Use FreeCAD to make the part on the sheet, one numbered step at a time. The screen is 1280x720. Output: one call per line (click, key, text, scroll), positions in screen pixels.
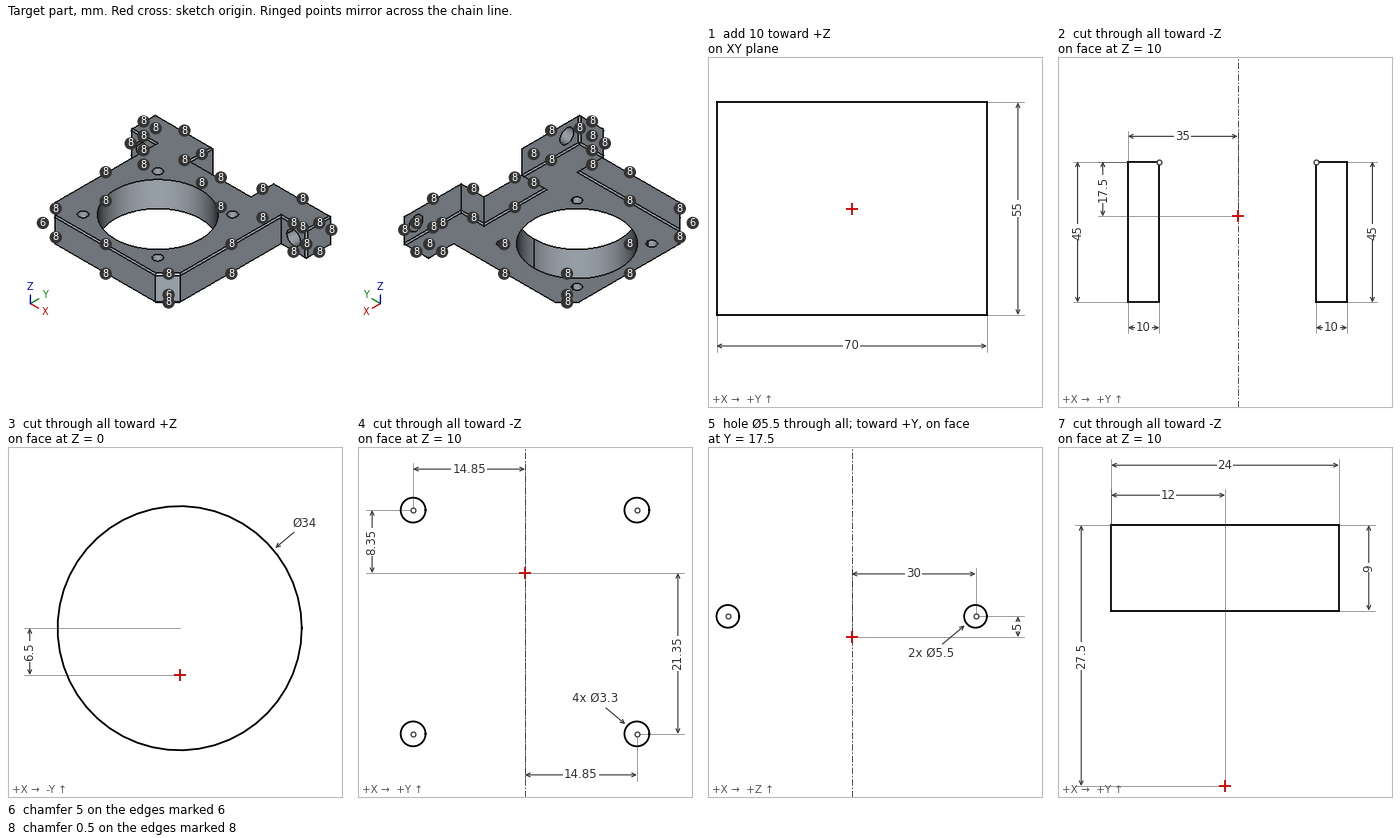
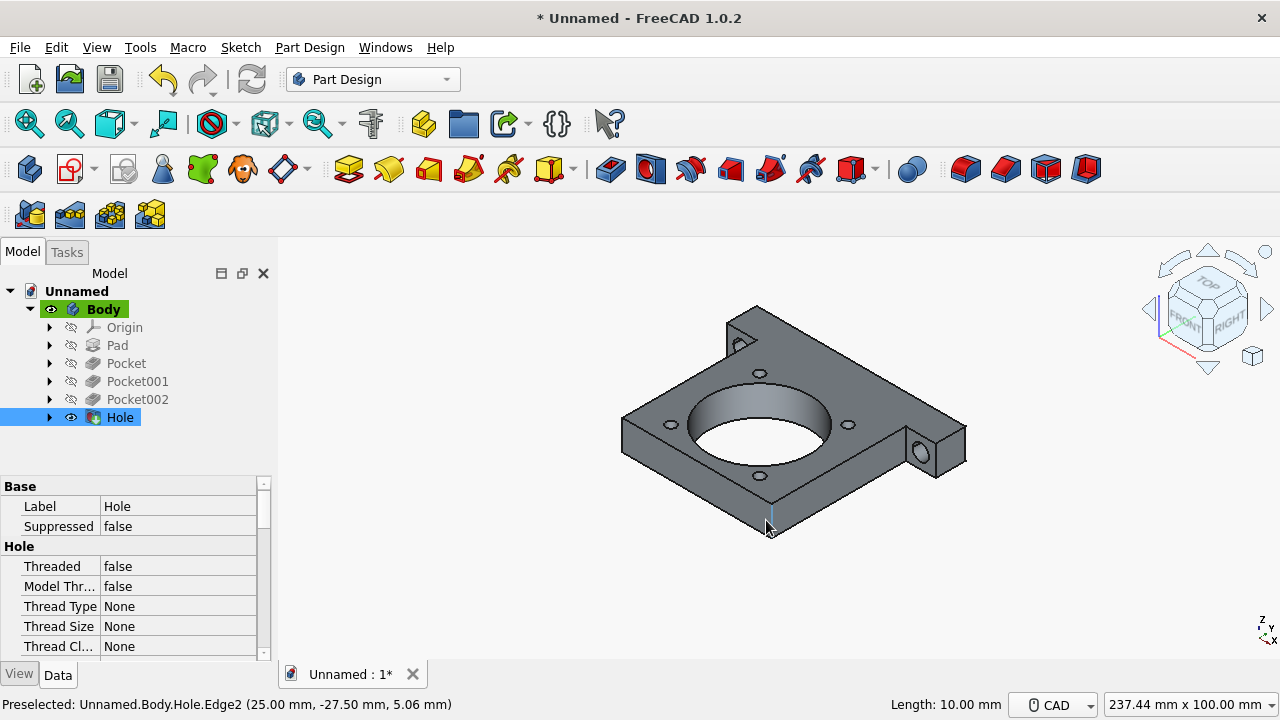
key(v)
key(f)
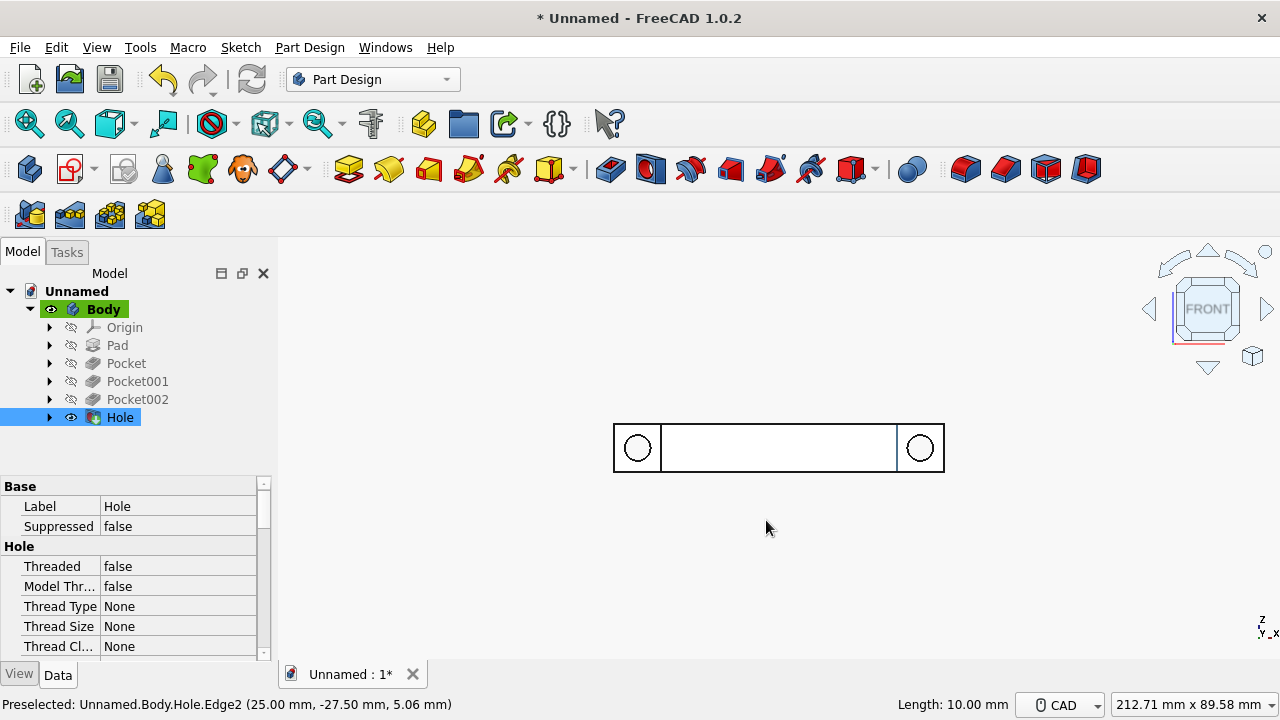
click(661, 447, ctrl)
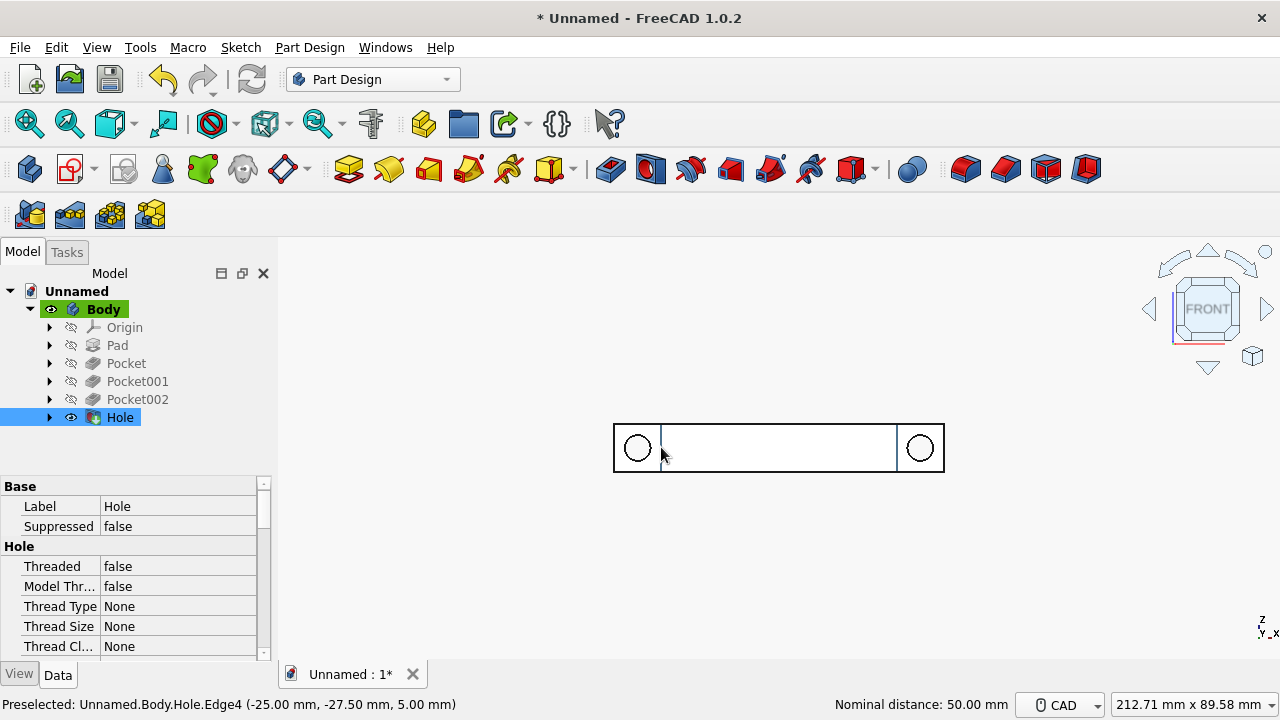
click(1006, 170)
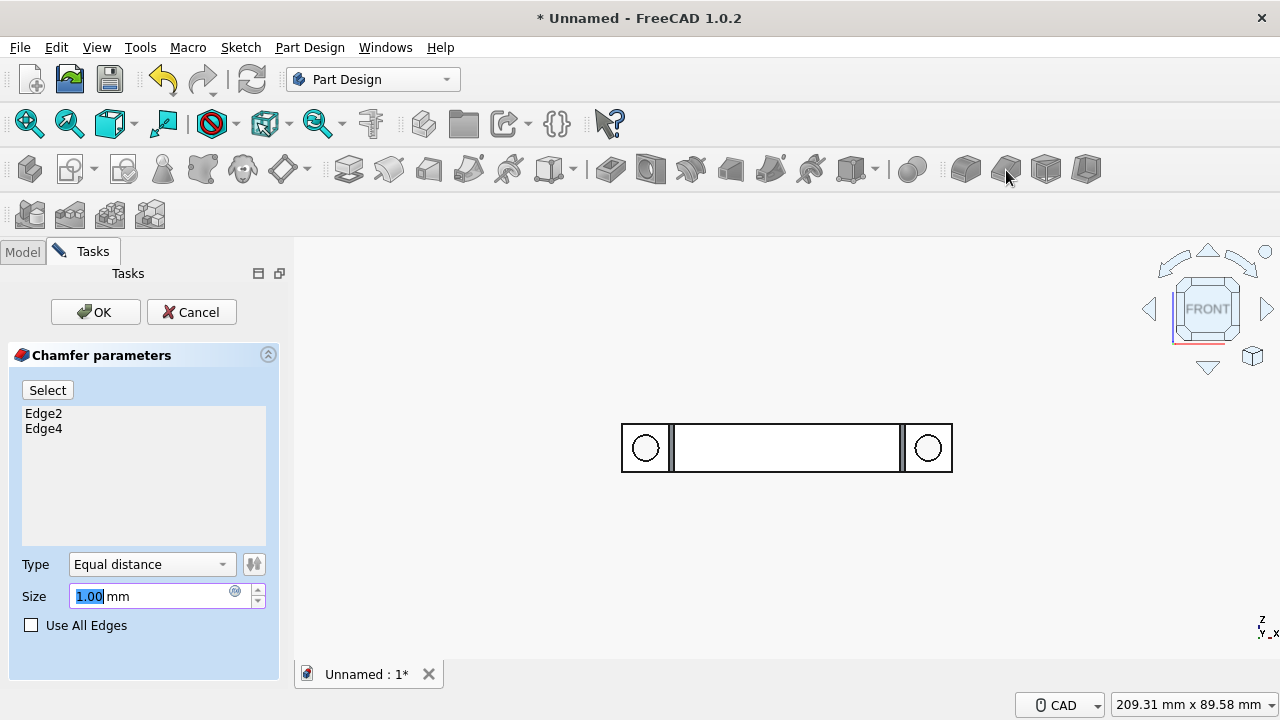
text(5)
key(Tab)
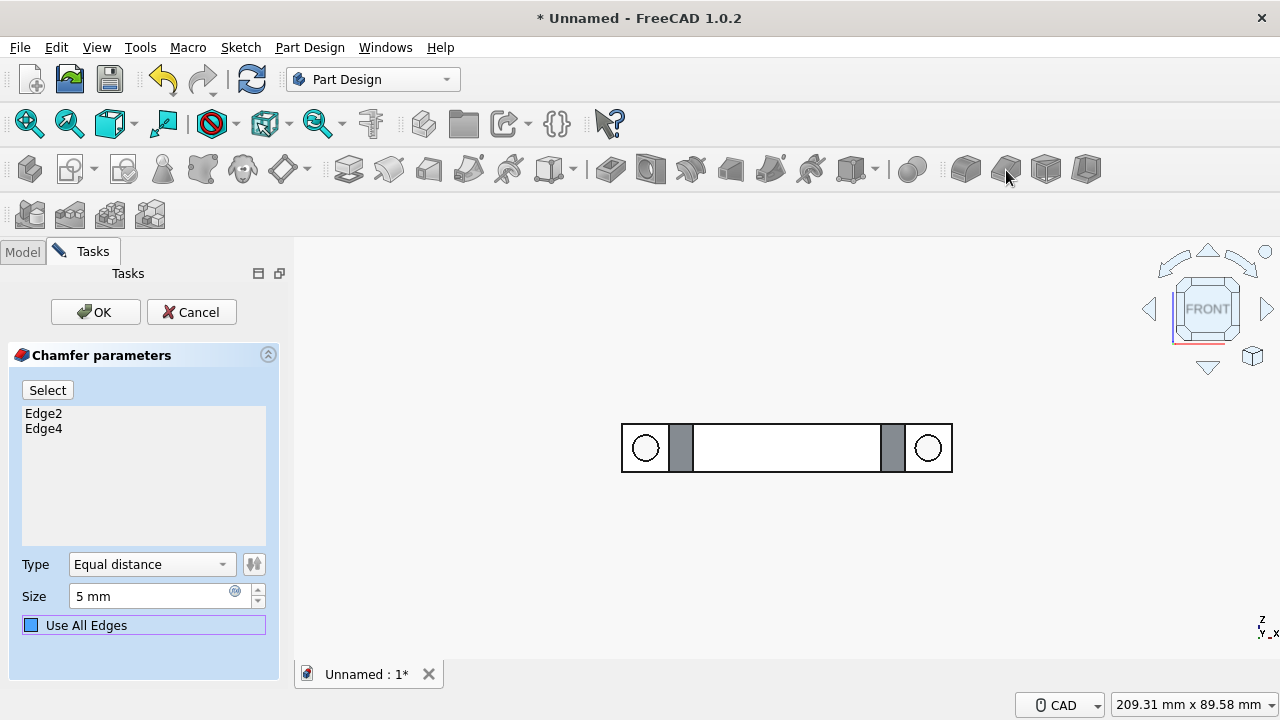
click(96, 312)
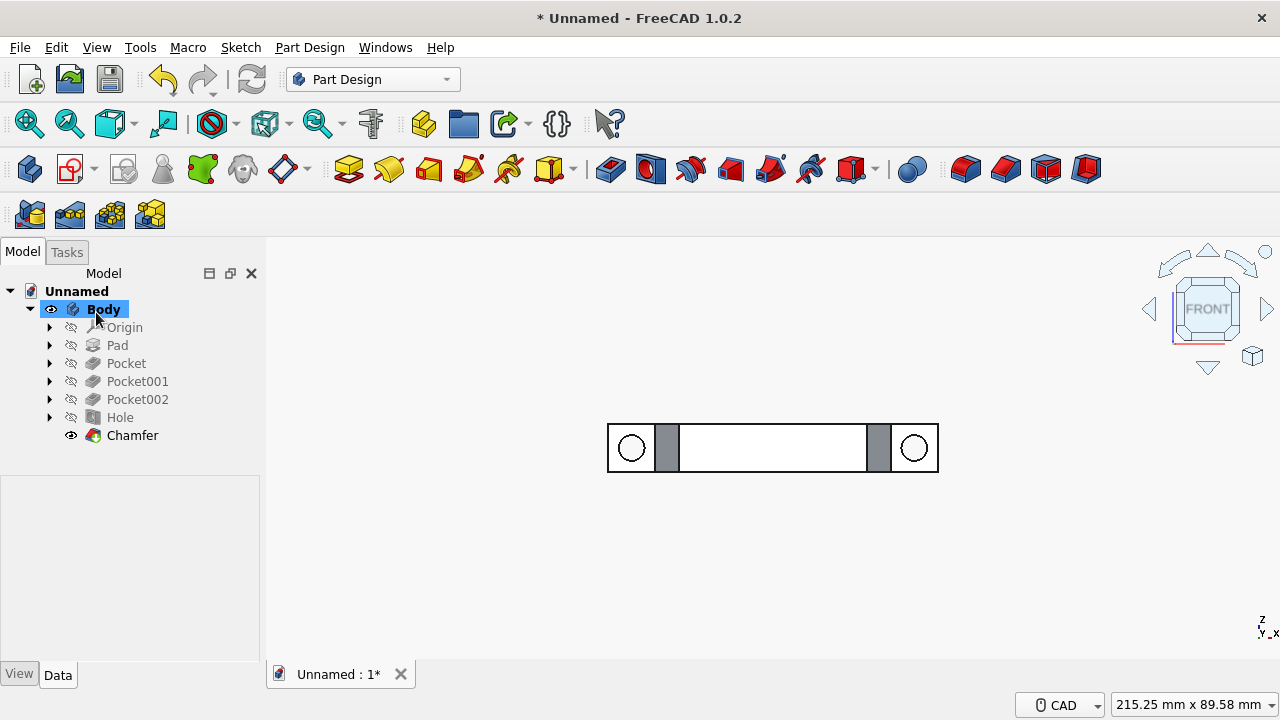
key(v)
key(f)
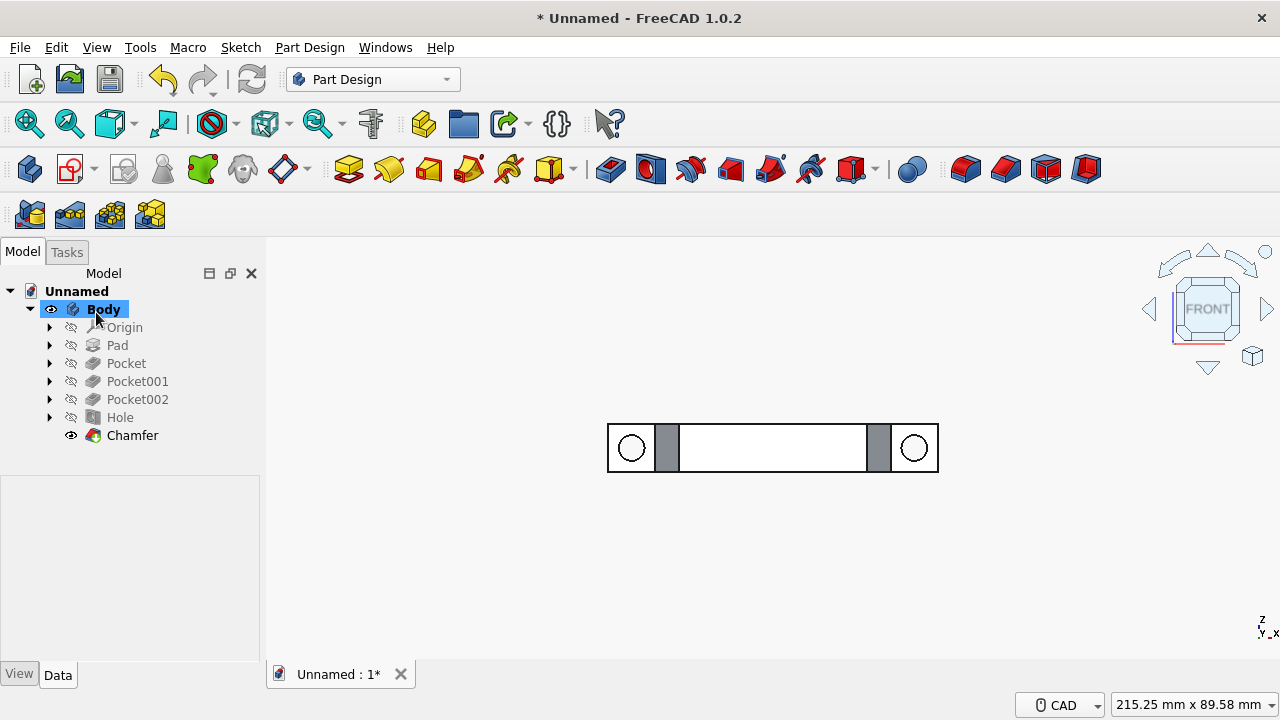
key(0)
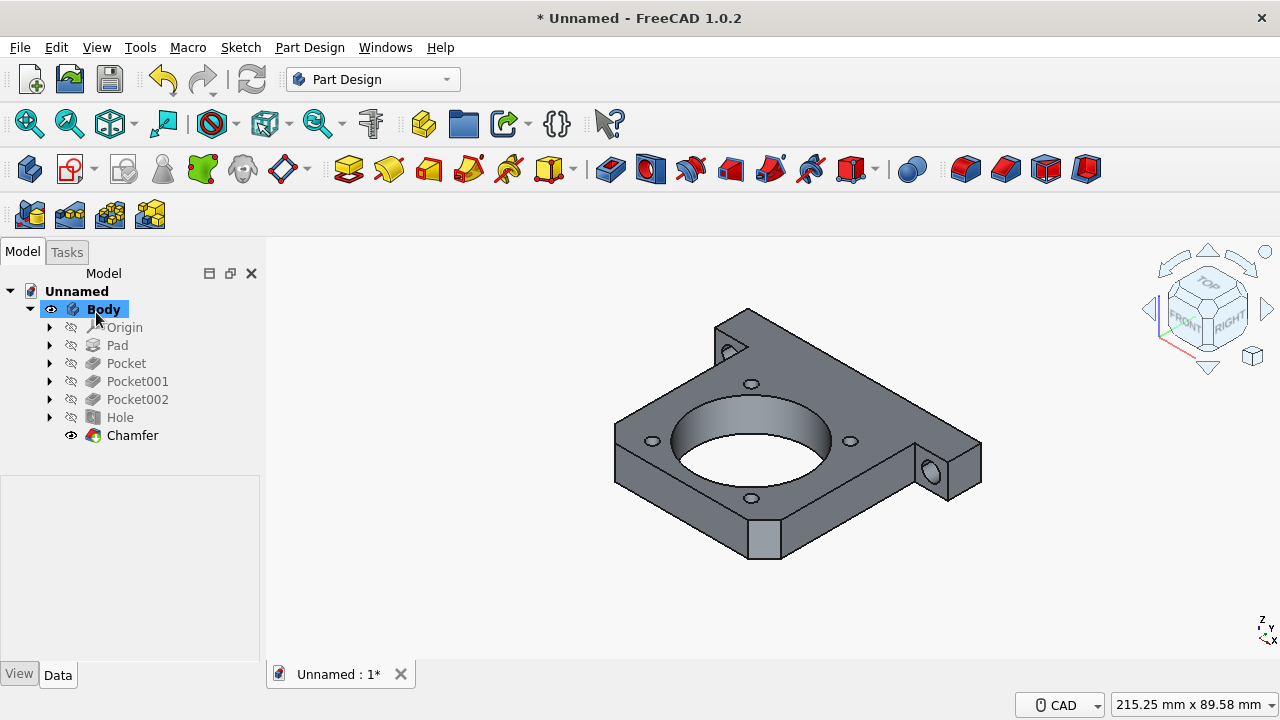
click(859, 417)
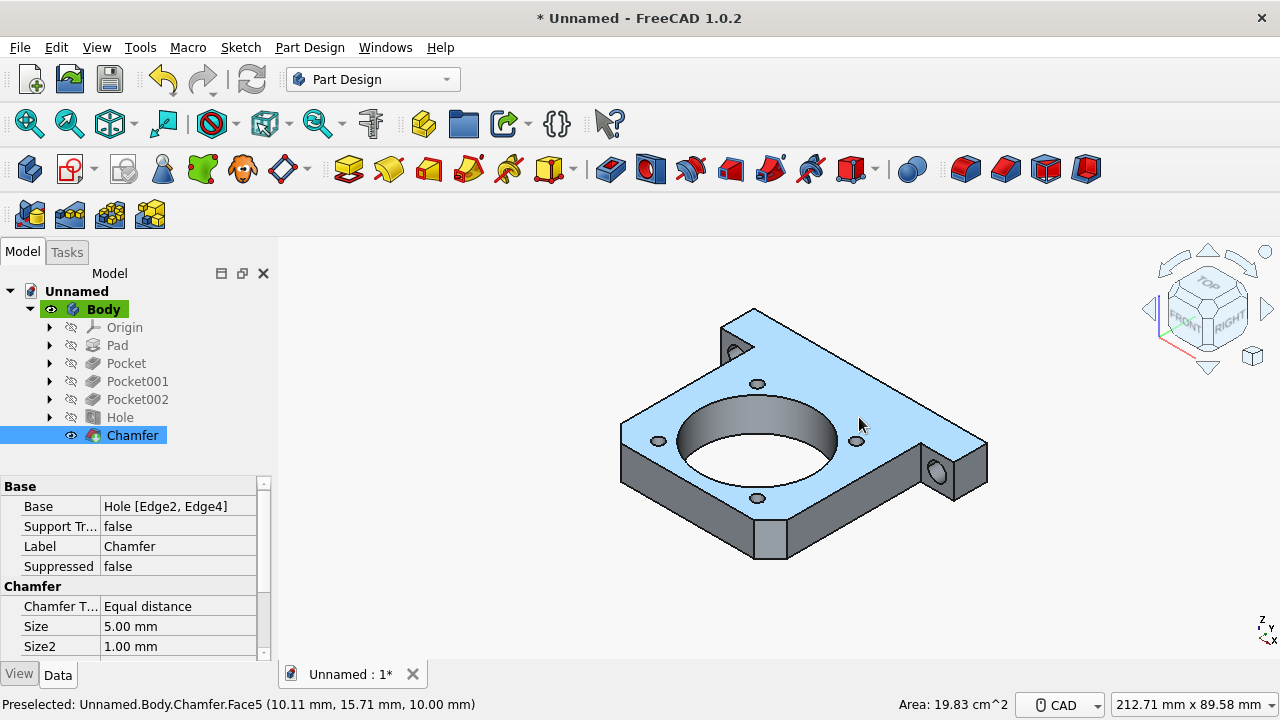
click(70, 170)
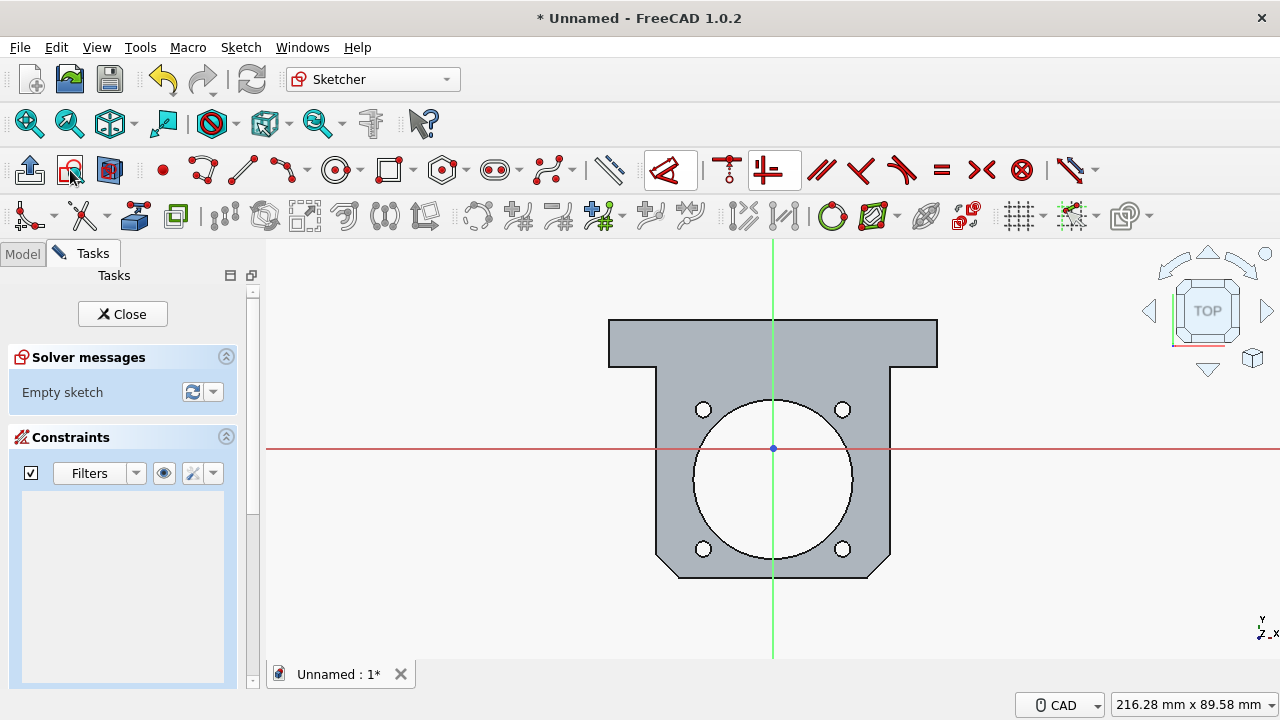
scroll(856, 306, up, 3)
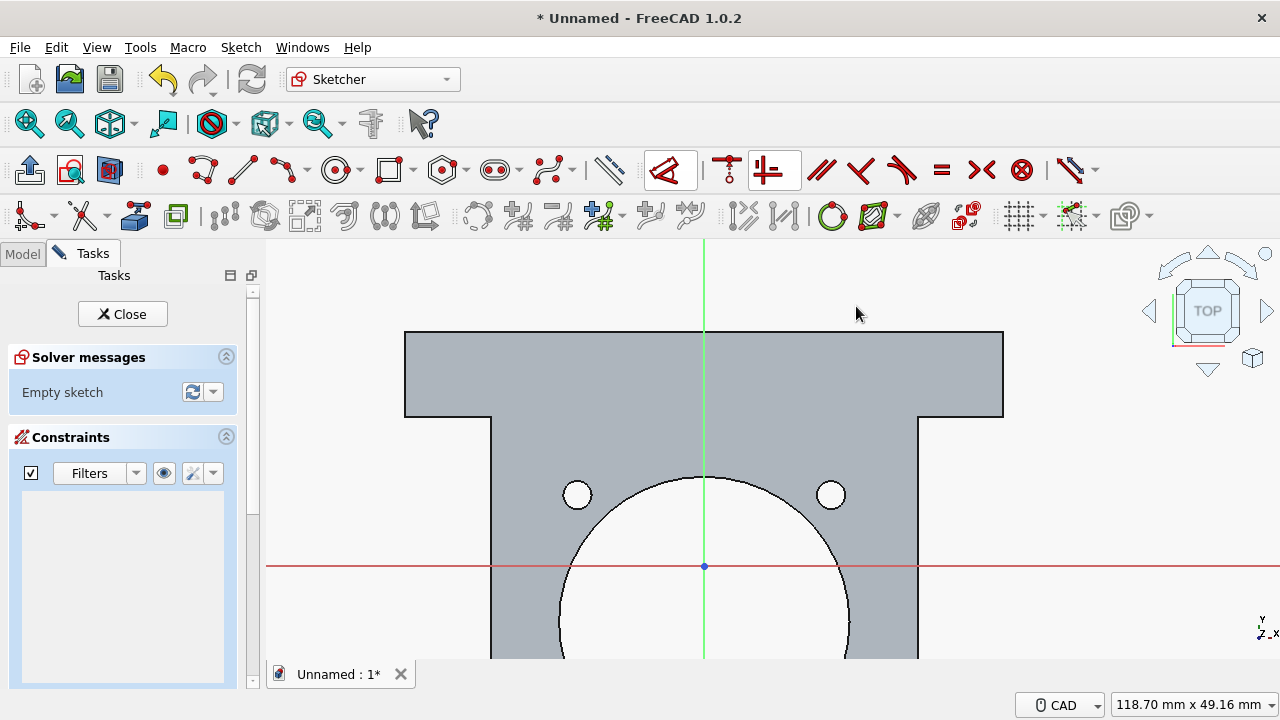
key(g)
key(r)